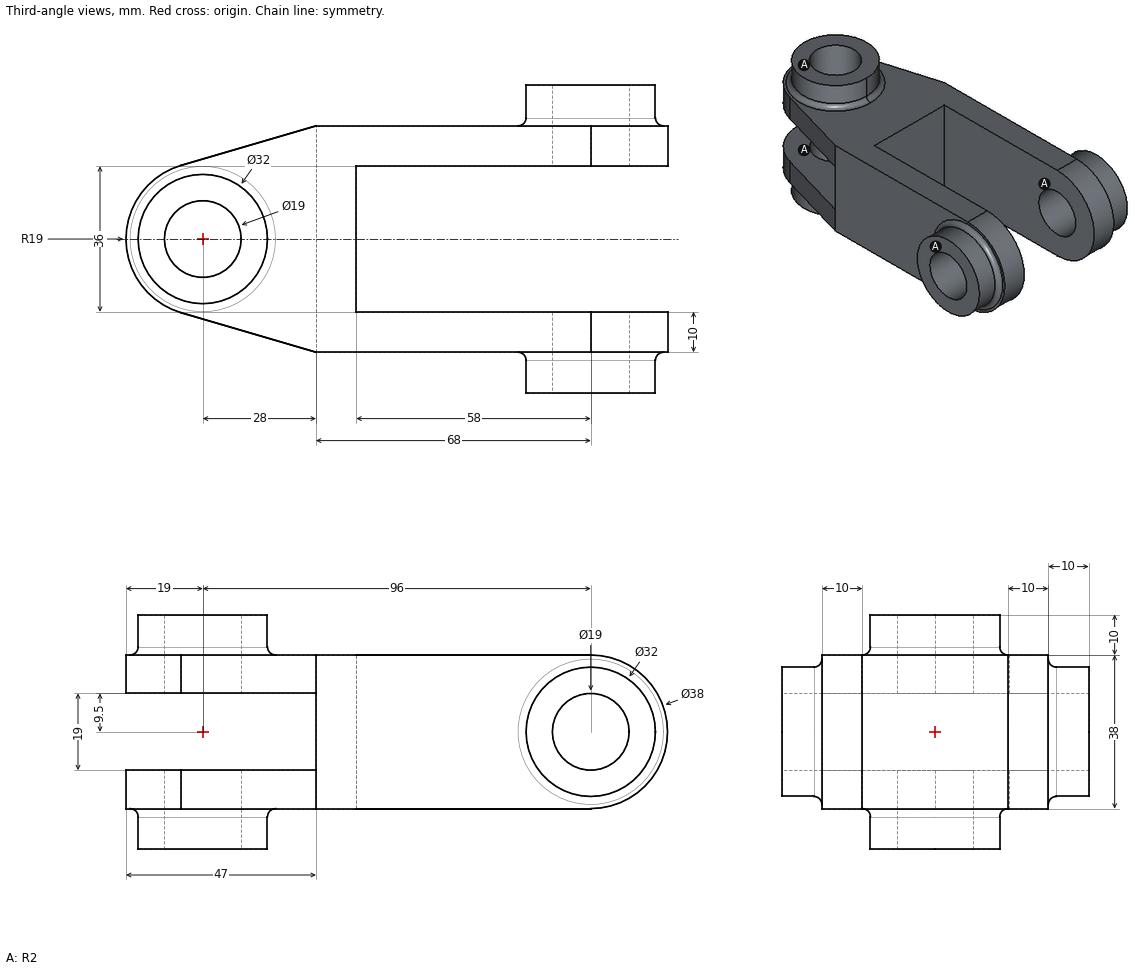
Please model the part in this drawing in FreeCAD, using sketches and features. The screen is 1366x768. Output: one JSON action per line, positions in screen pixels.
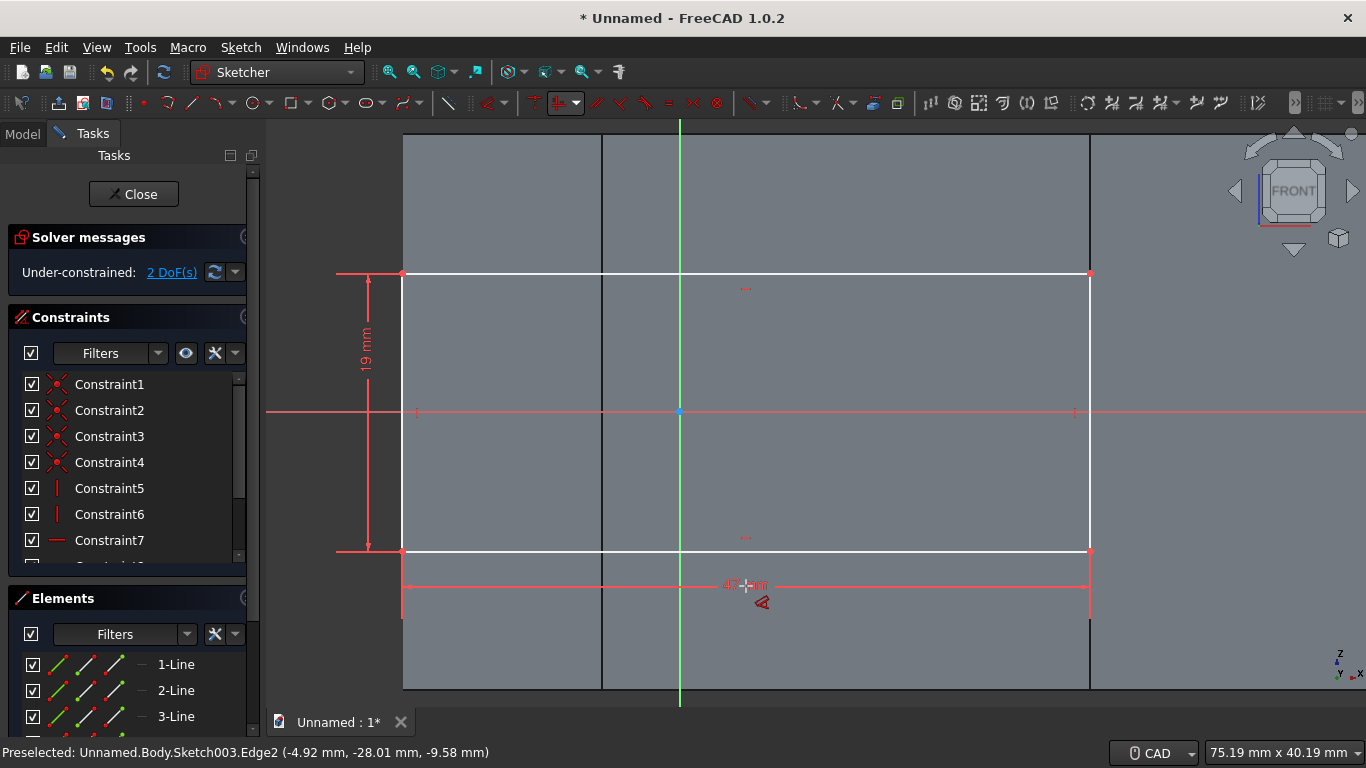
{"action": "left_click", "coordinate": [402, 274]}
{"action": "left_click", "coordinate": [541, 240]}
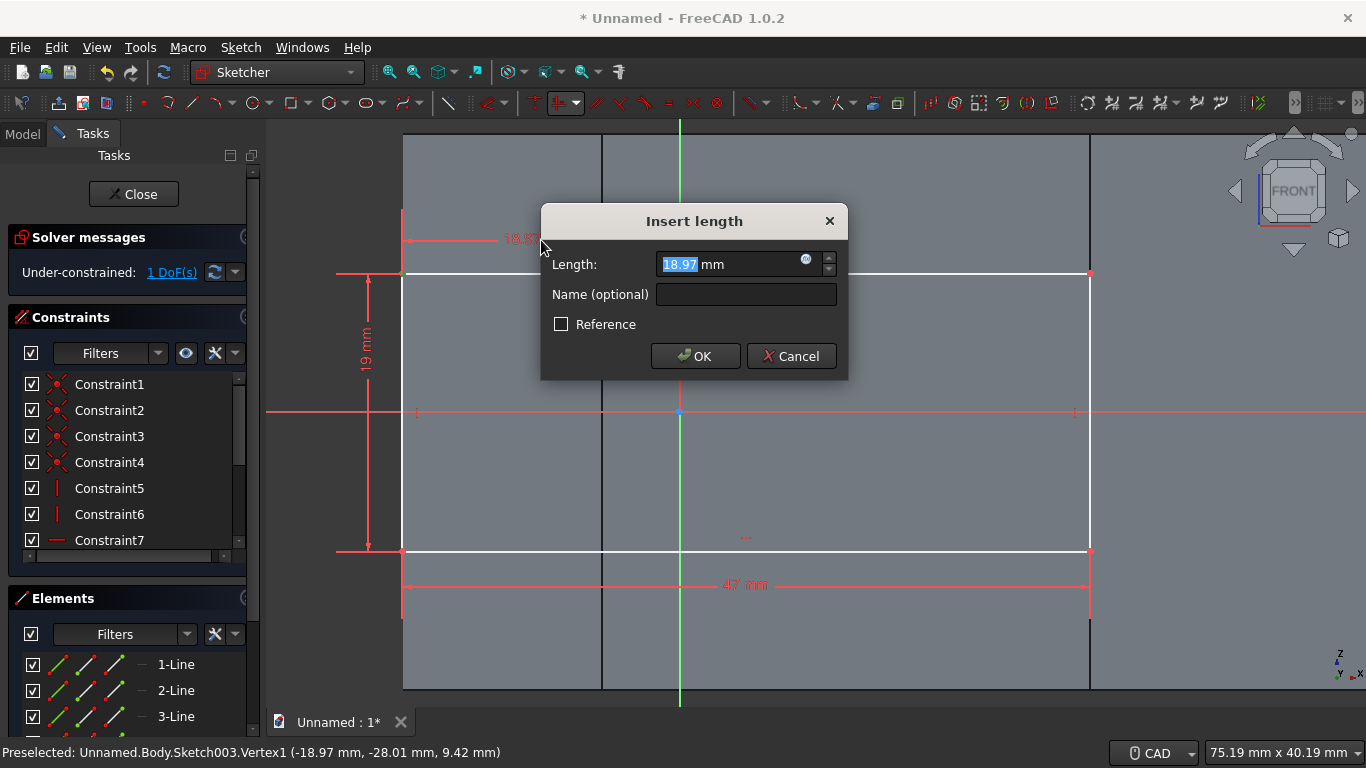
{"action": "type", "text": "19"}
{"action": "key", "text": "Return"}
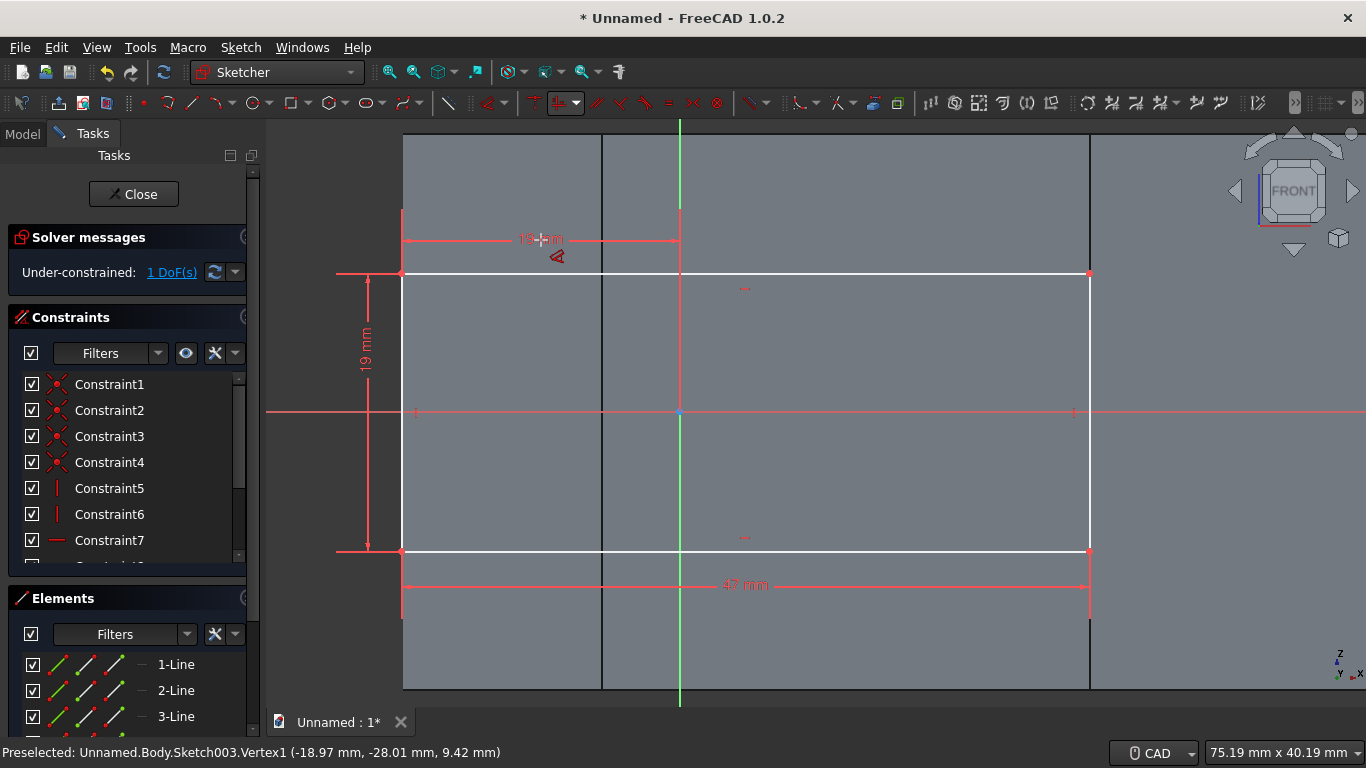
{"action": "left_click", "coordinate": [402, 274]}
{"action": "left_click", "coordinate": [368, 311]}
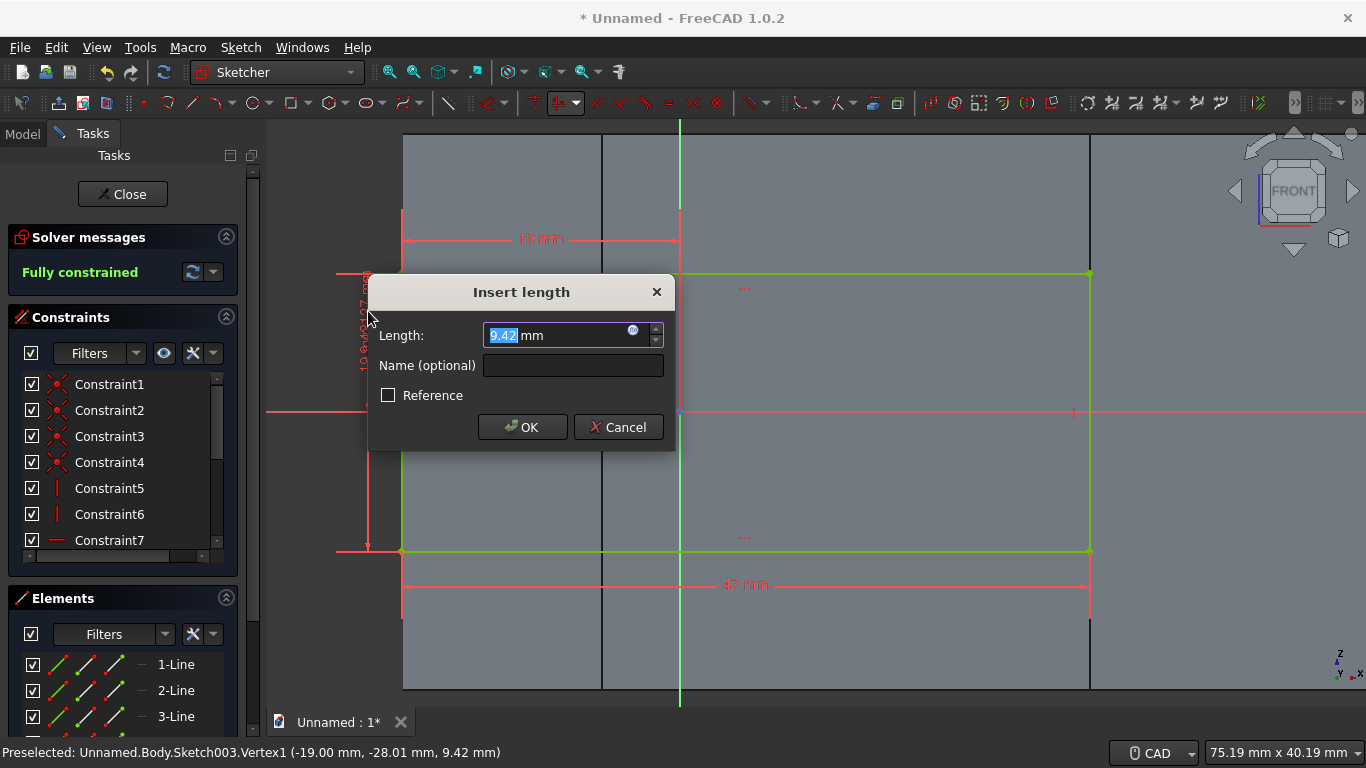
{"action": "type", "text": "9.5"}
{"action": "key", "text": "Return"}
{"action": "key", "text": "Escape"}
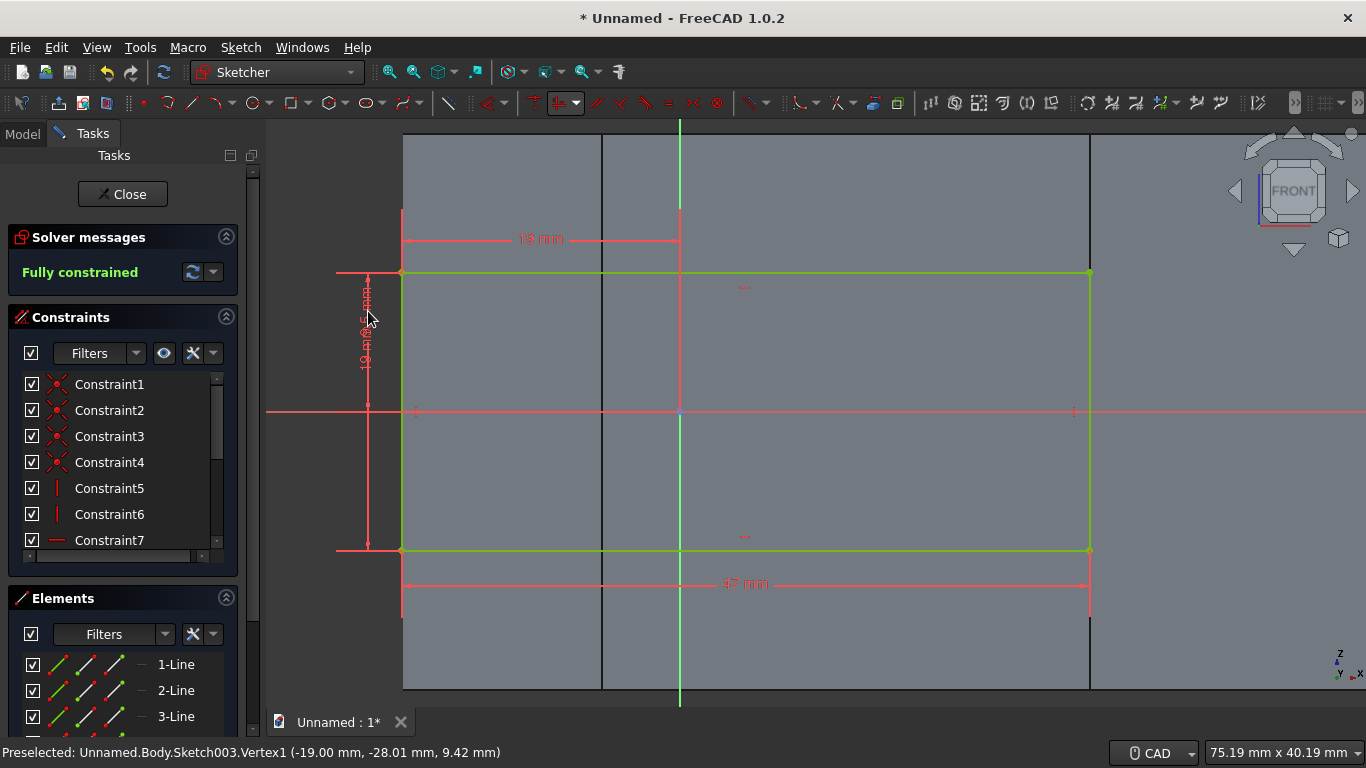
{"action": "left_click", "coordinate": [123, 194]}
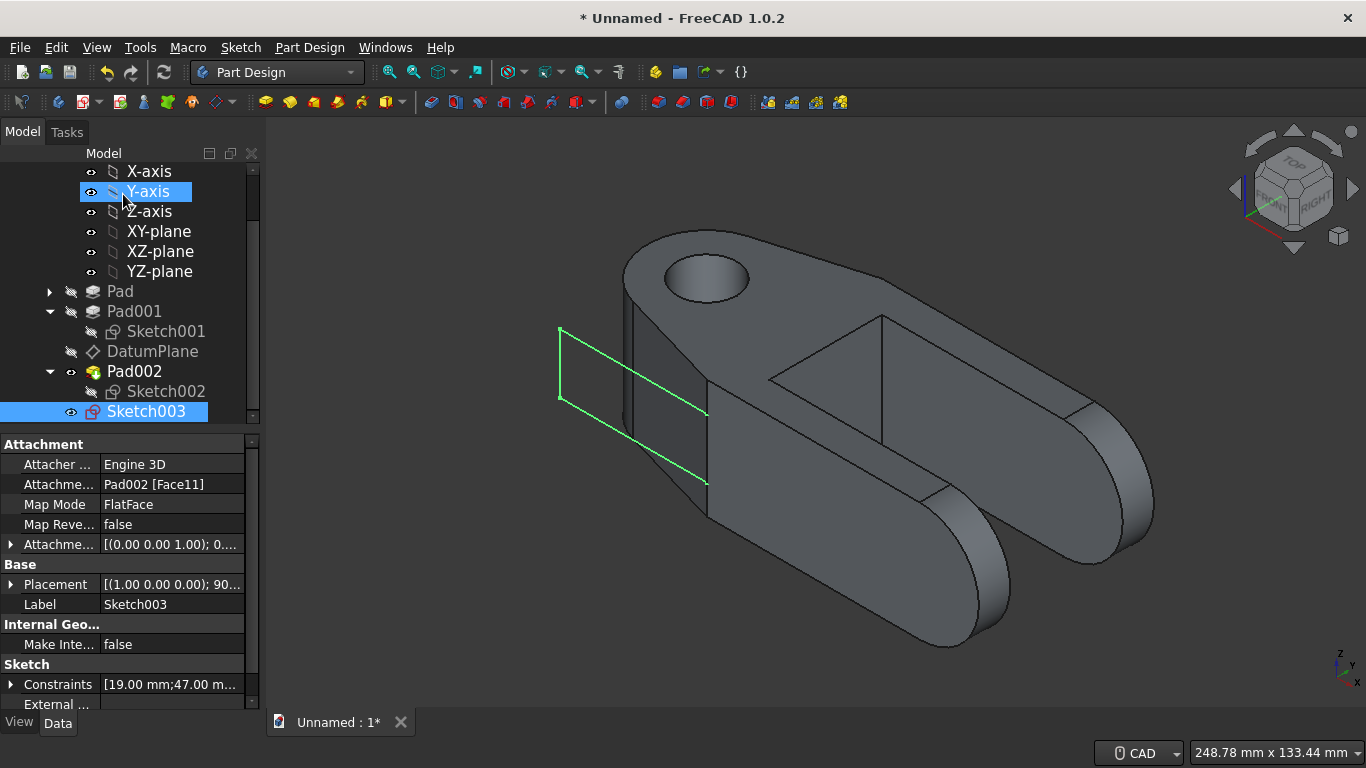
{"action": "left_click", "coordinate": [432, 102]}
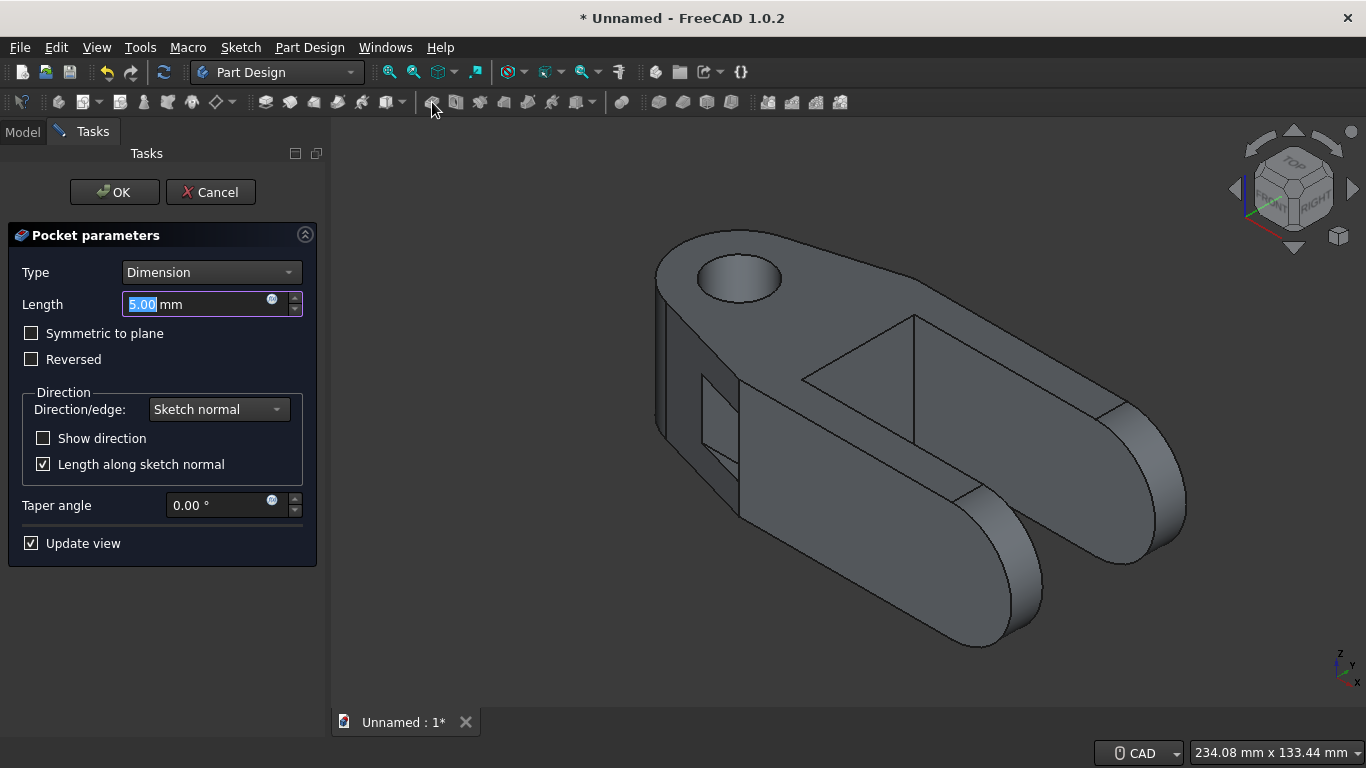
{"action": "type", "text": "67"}
{"action": "key", "text": "Tab"}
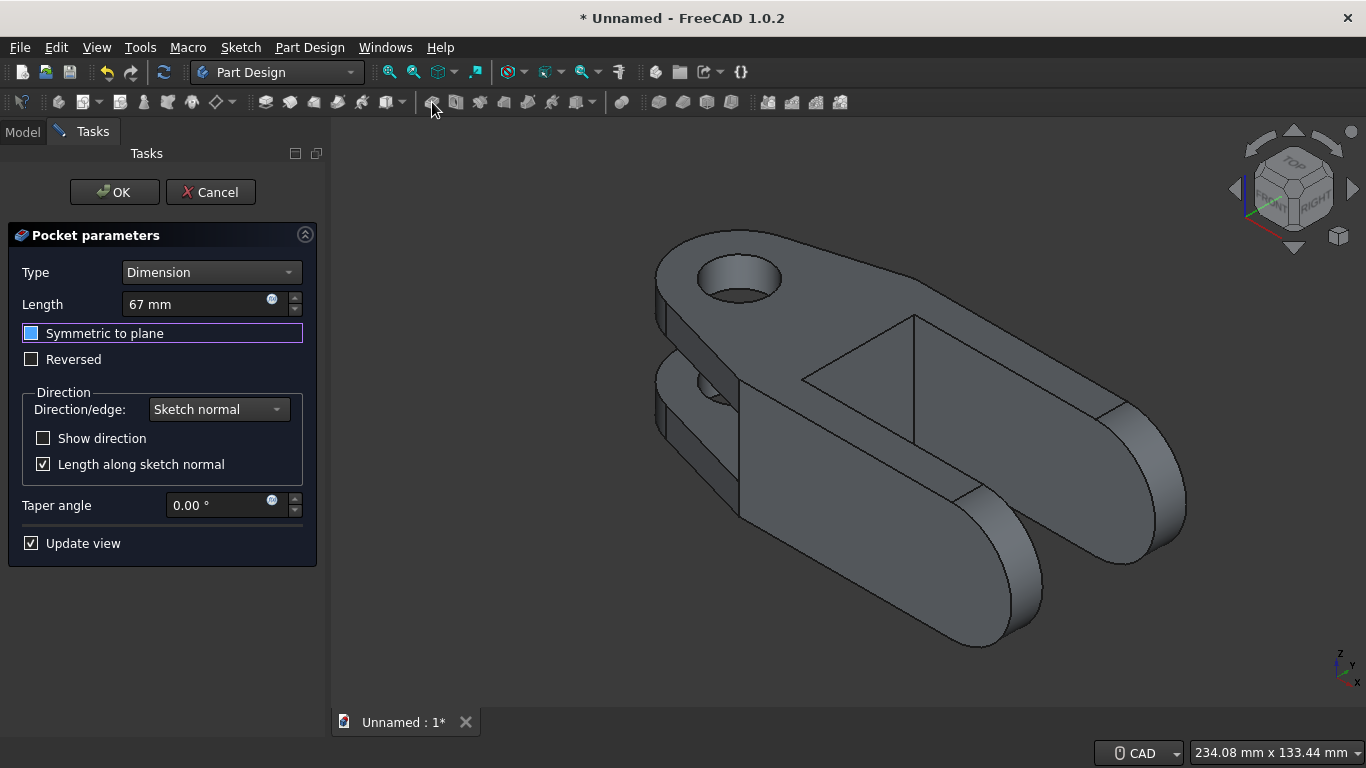
{"action": "left_click", "coordinate": [115, 192]}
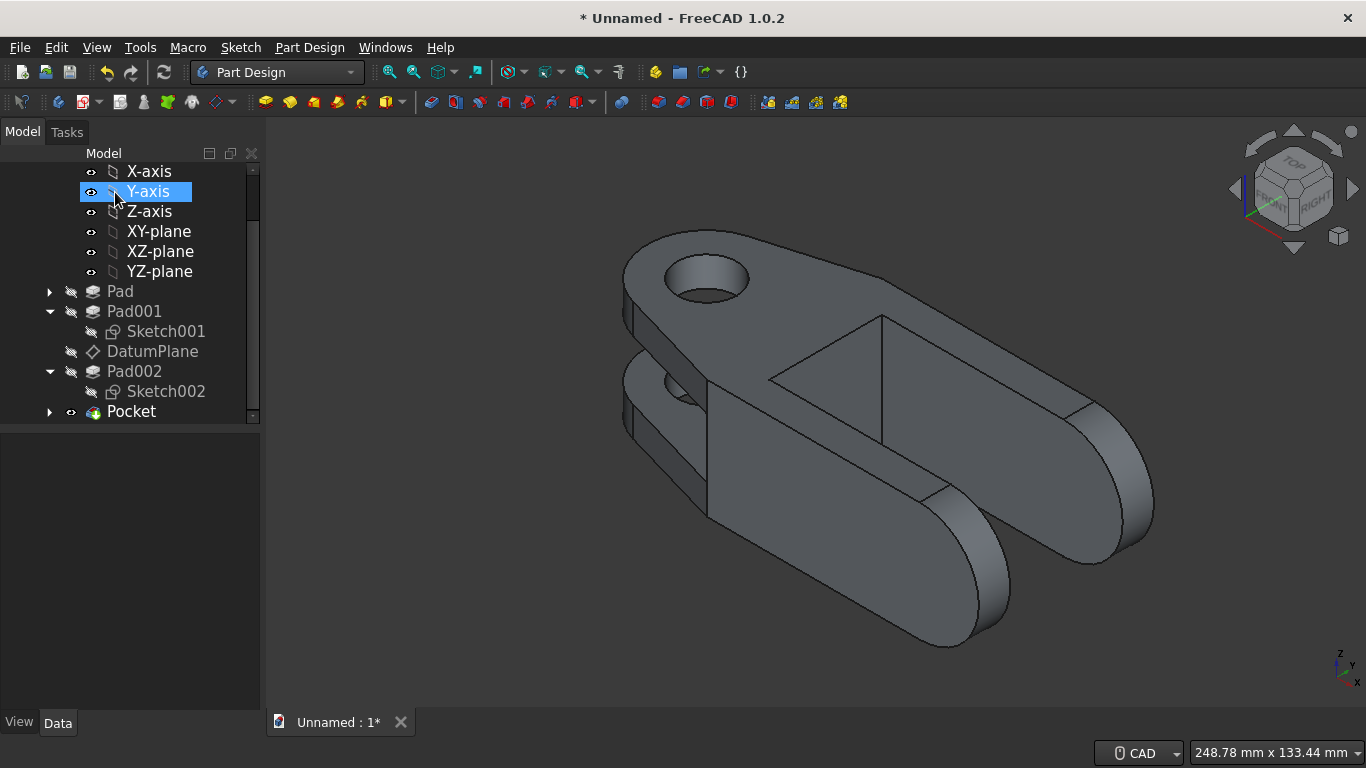
{"action": "left_click", "coordinate": [801, 303]}